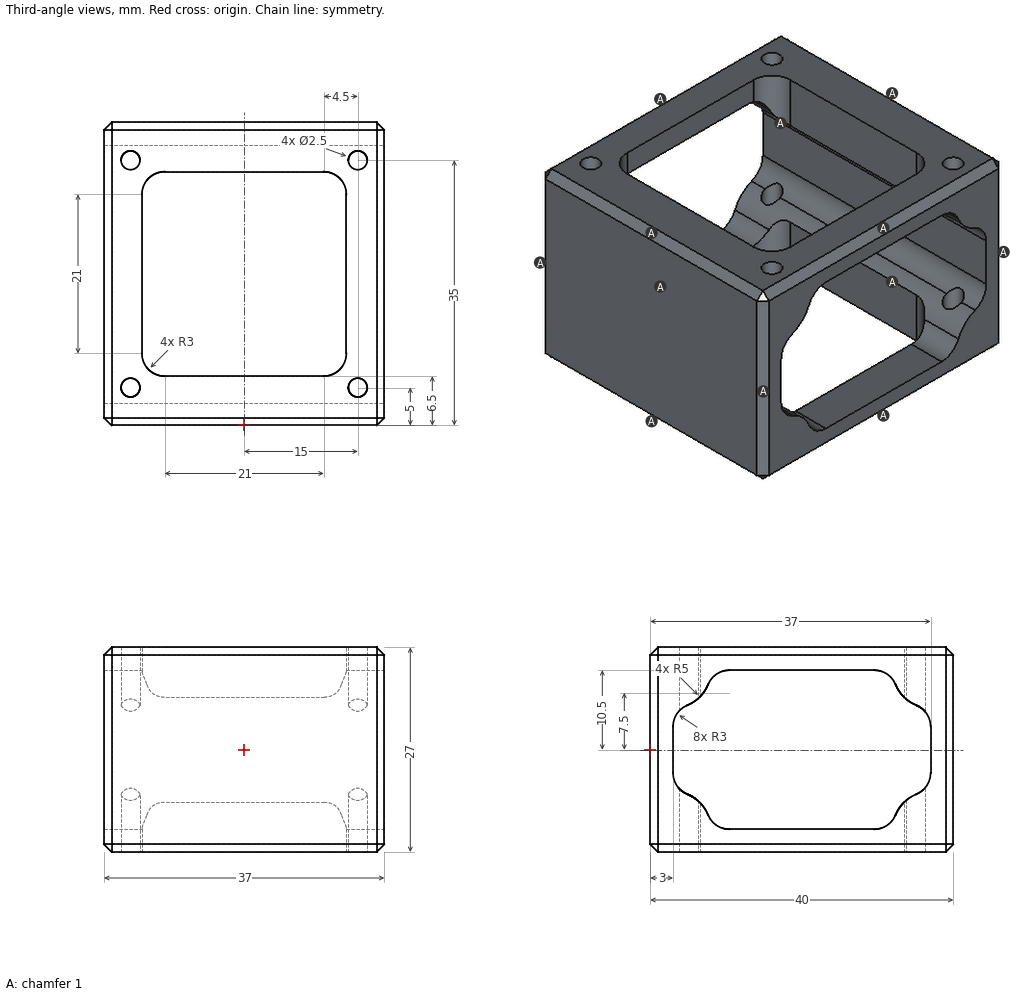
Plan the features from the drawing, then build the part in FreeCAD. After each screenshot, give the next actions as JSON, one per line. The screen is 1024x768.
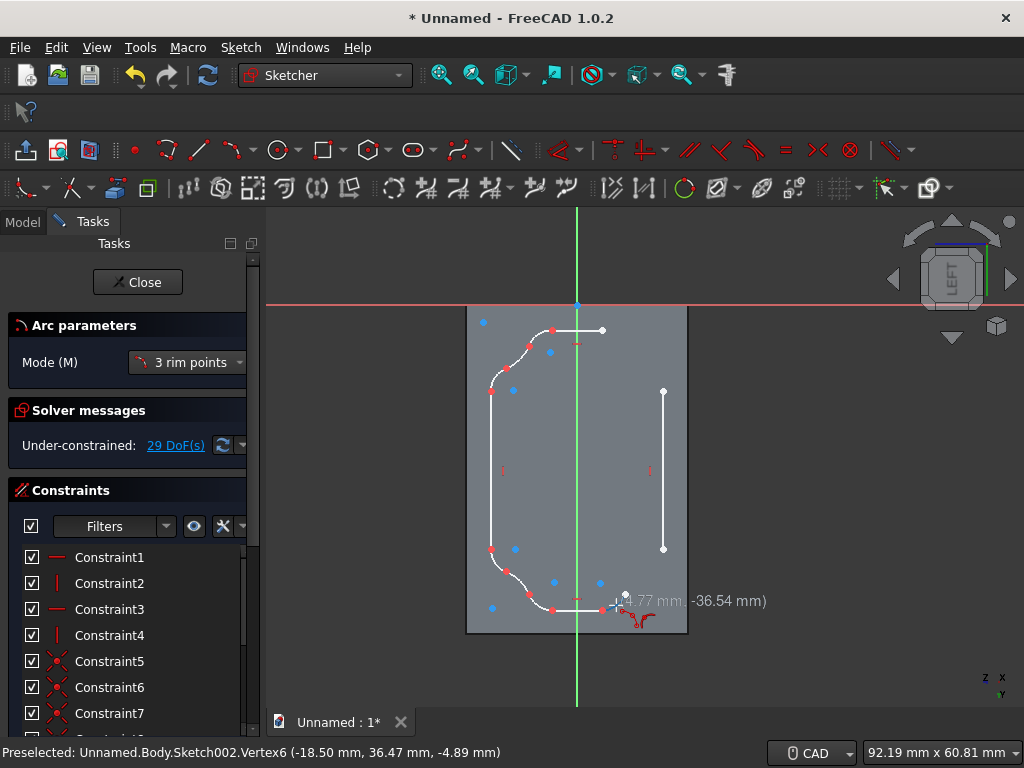
{"action": "left_click", "coordinate": [625, 595]}
{"action": "left_click", "coordinate": [648, 571]}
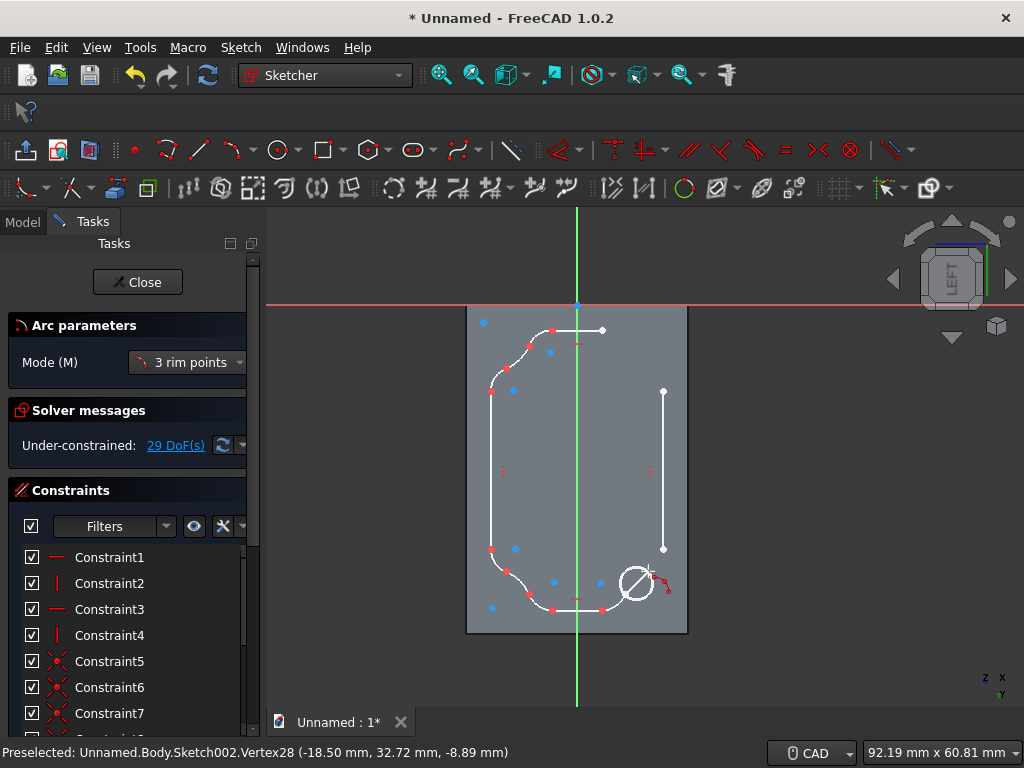
{"action": "scroll", "coordinate": [634, 581], "scroll_direction": "up", "scroll_amount": 8}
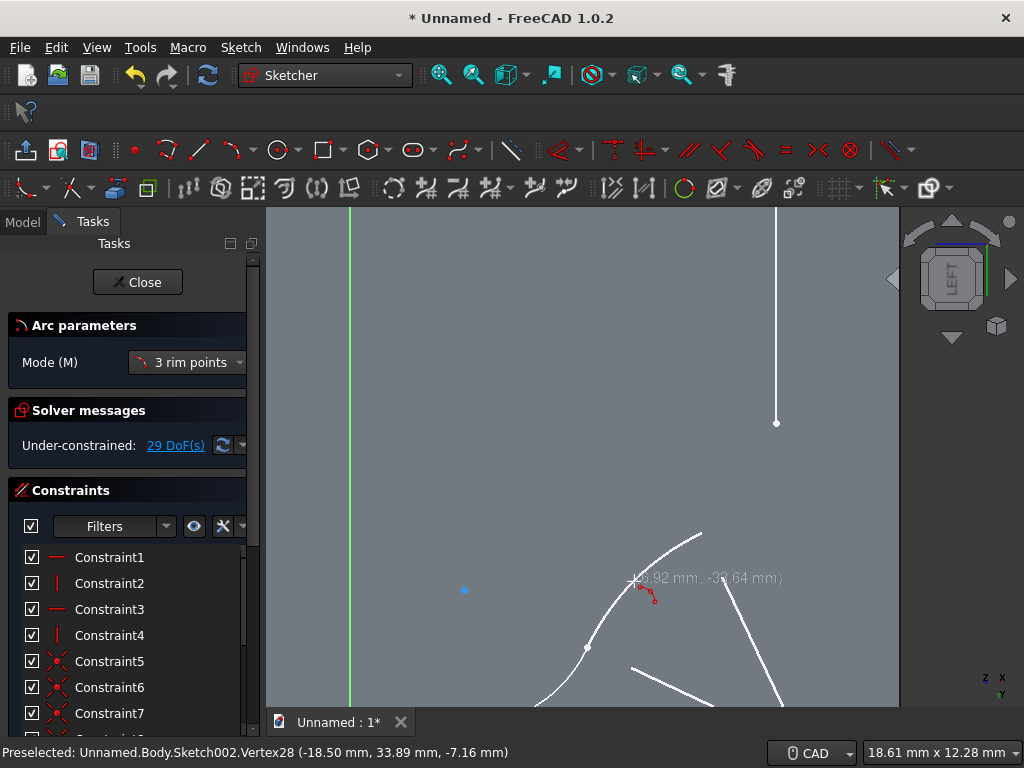
{"action": "left_click", "coordinate": [634, 576]}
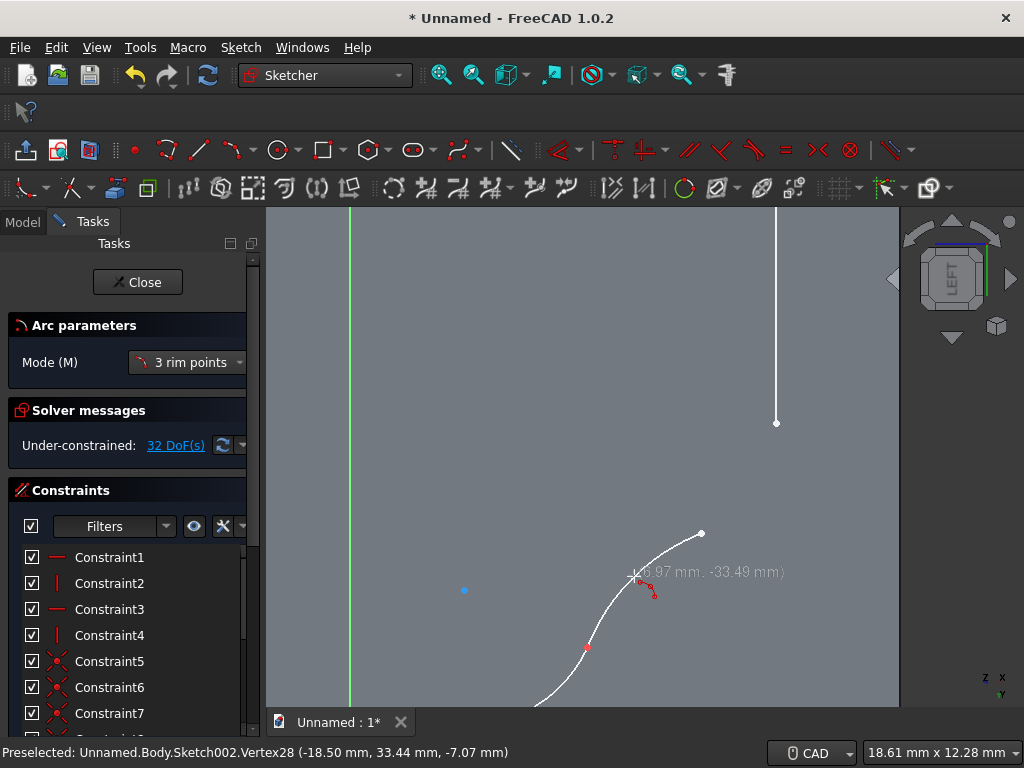
{"action": "scroll", "coordinate": [634, 581], "scroll_direction": "down", "scroll_amount": 8}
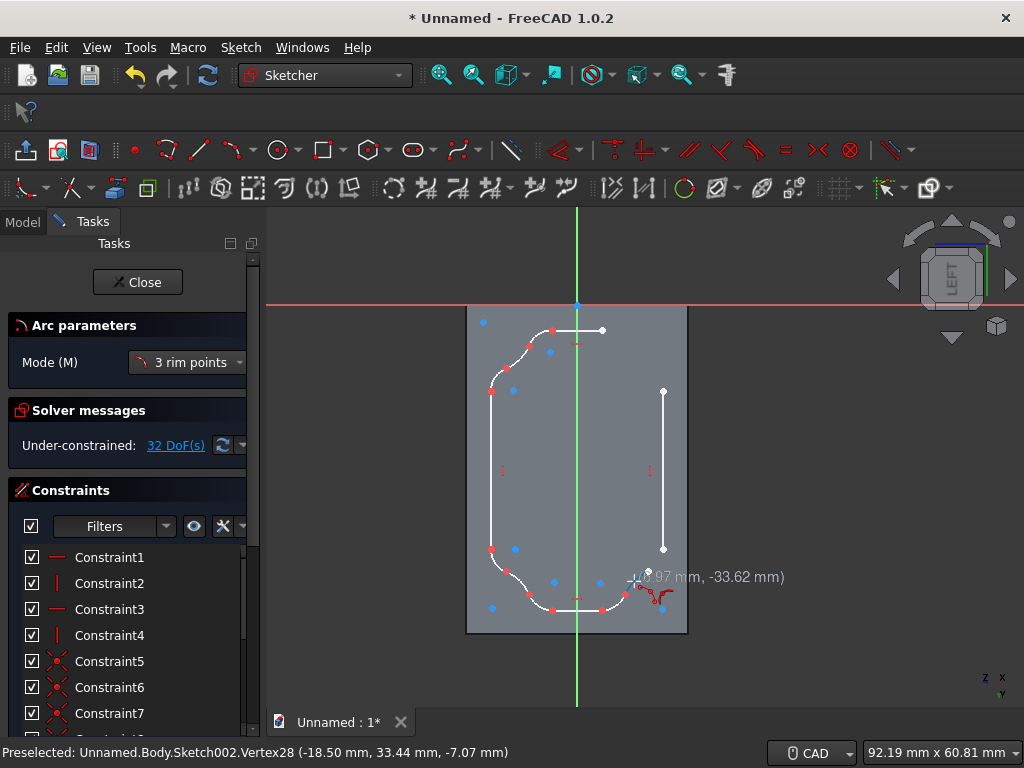
{"action": "left_click", "coordinate": [648, 572]}
{"action": "left_click", "coordinate": [663, 550]}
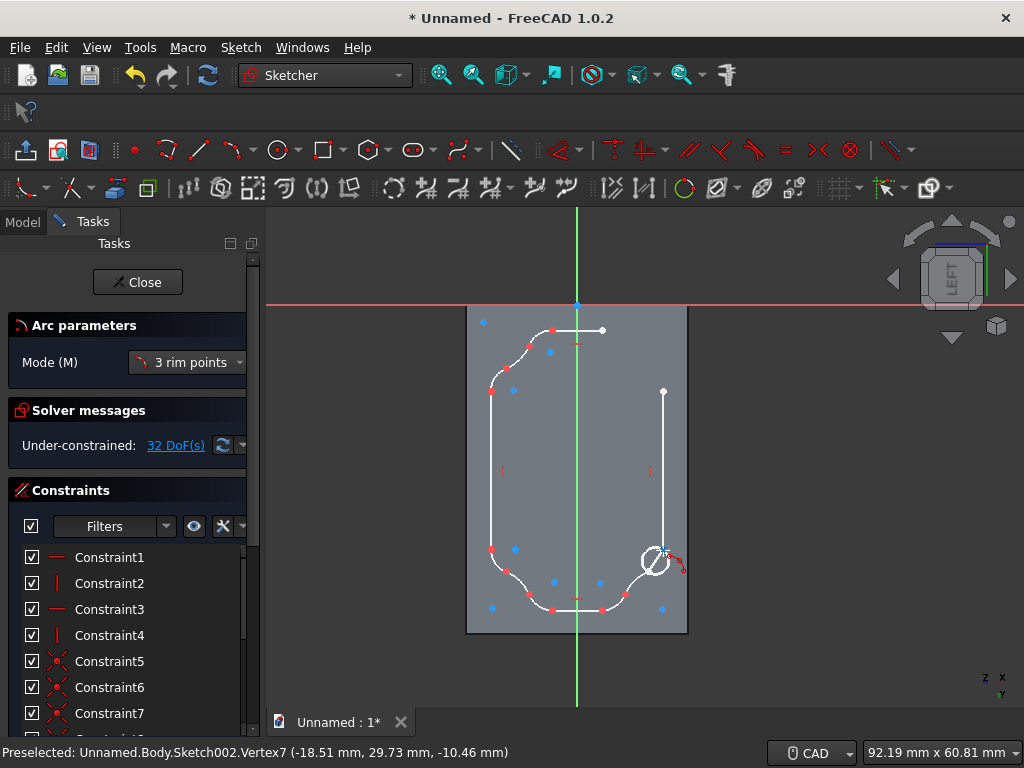
{"action": "scroll", "coordinate": [659, 562], "scroll_direction": "up", "scroll_amount": 7}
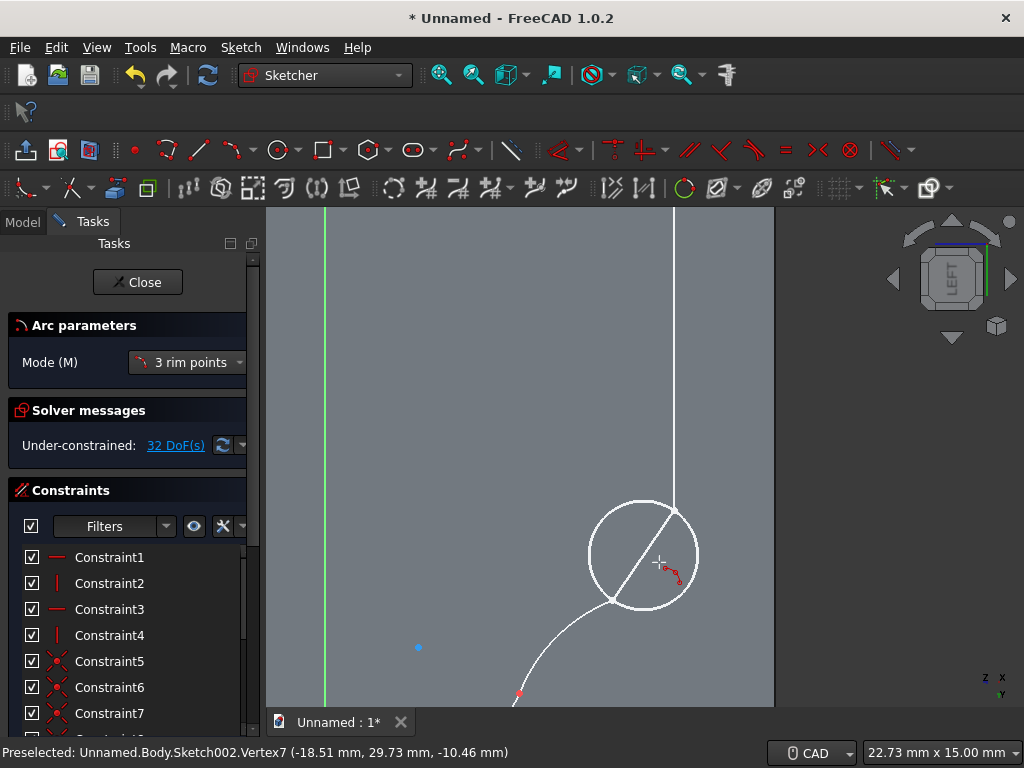
{"action": "left_click", "coordinate": [658, 562]}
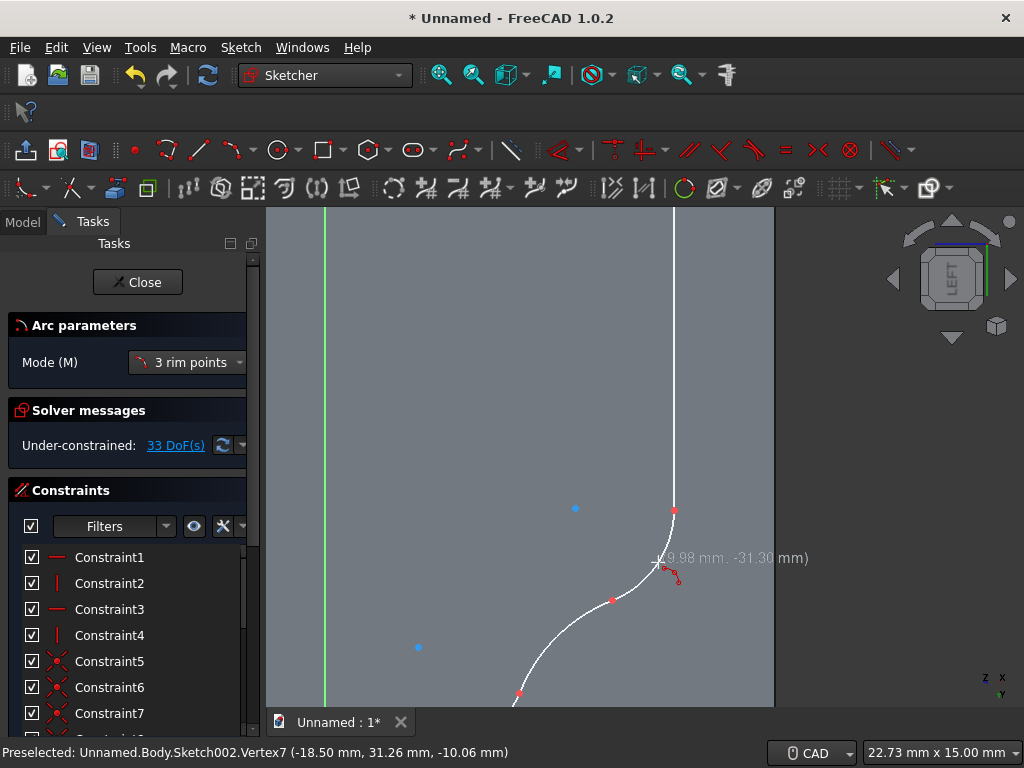
{"action": "scroll", "coordinate": [659, 562], "scroll_direction": "down", "scroll_amount": 7}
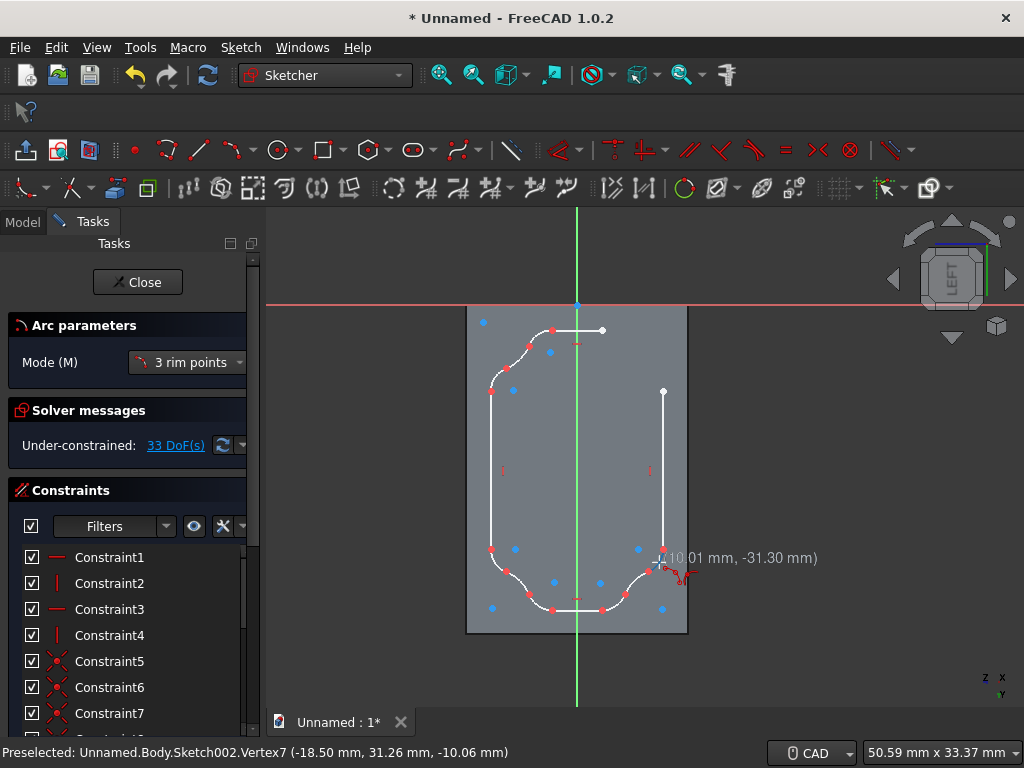
{"action": "left_click", "coordinate": [663, 392]}
{"action": "left_click", "coordinate": [648, 368]}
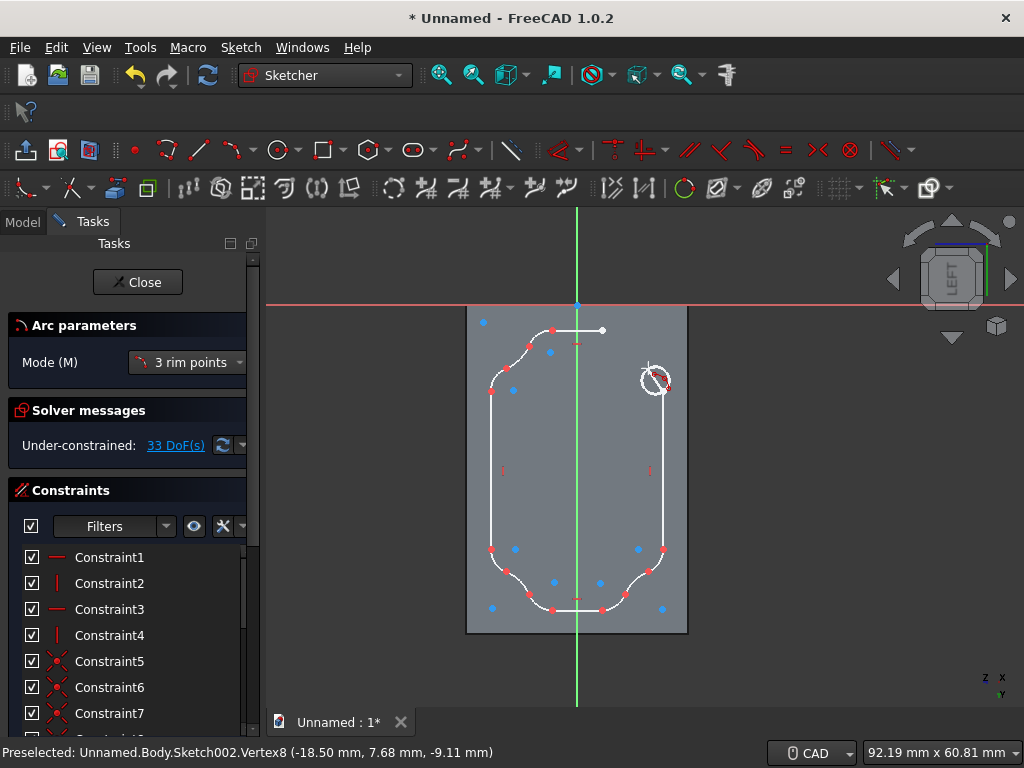
{"action": "scroll", "coordinate": [659, 377], "scroll_direction": "up", "scroll_amount": 7}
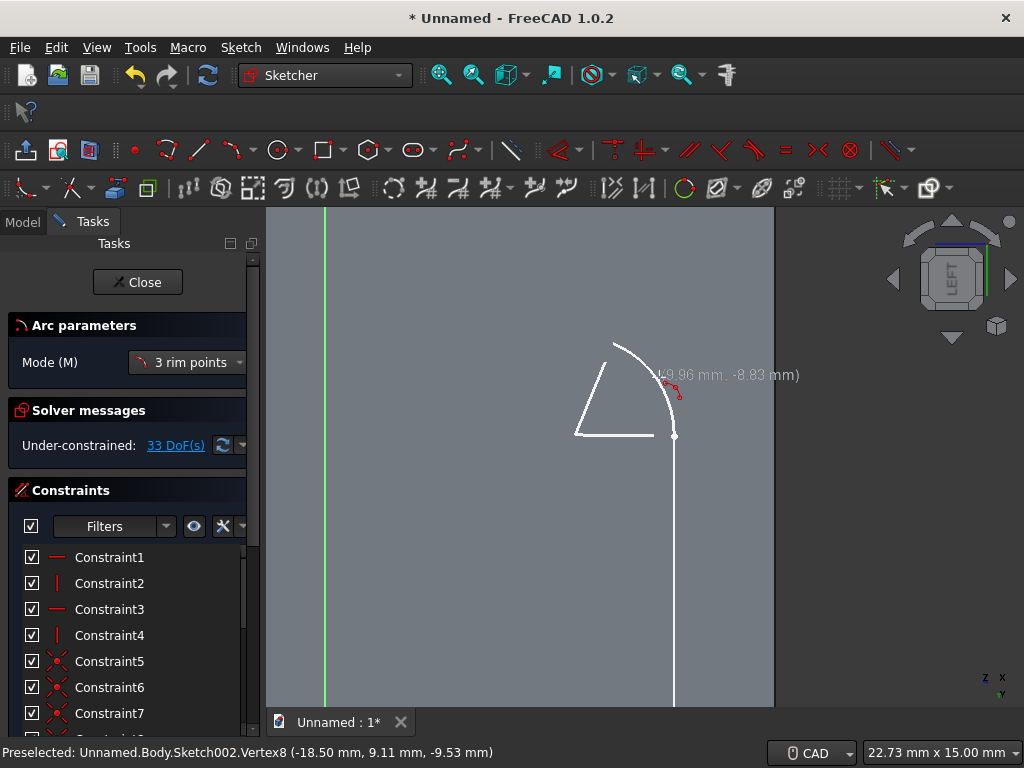
{"action": "left_click", "coordinate": [658, 377]}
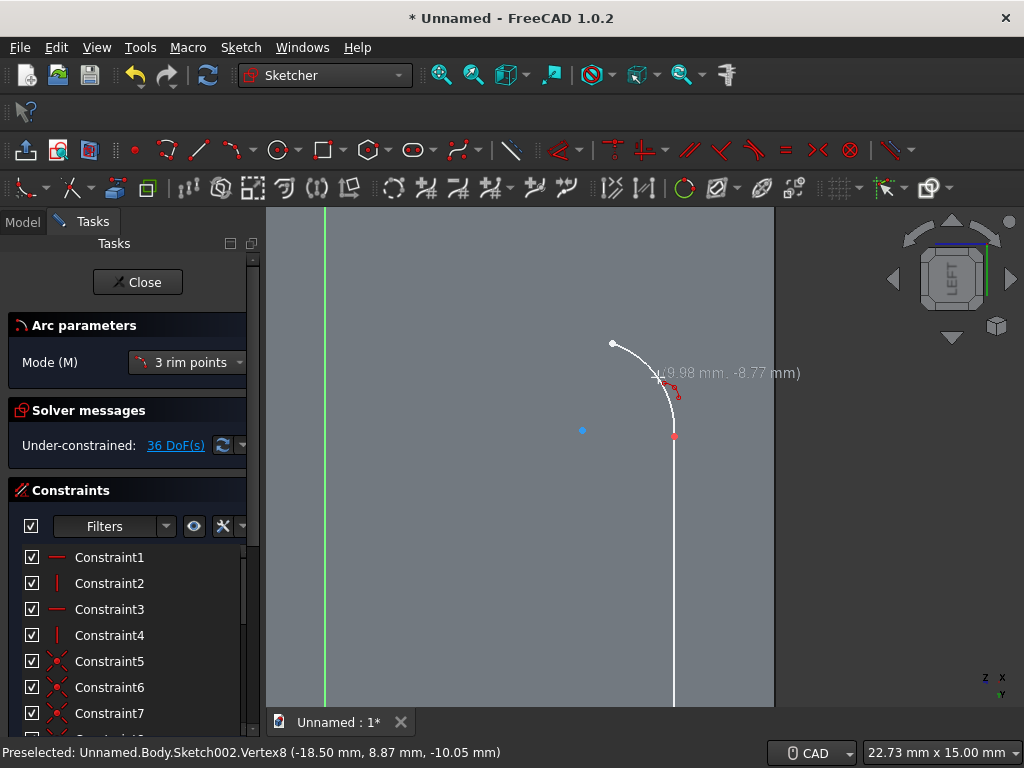
{"action": "scroll", "coordinate": [659, 377], "scroll_direction": "down", "scroll_amount": 7}